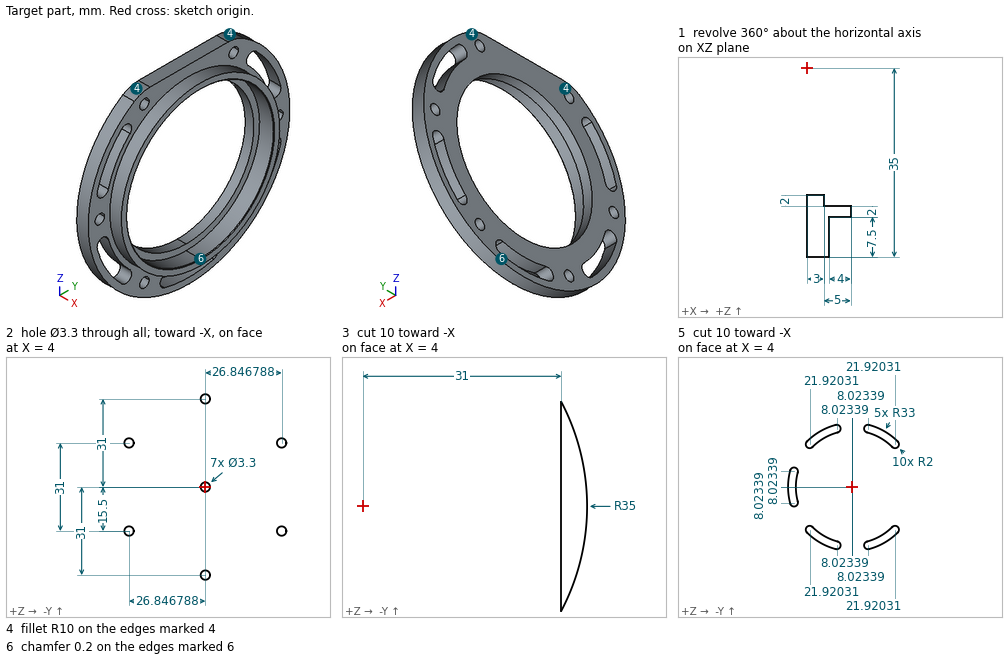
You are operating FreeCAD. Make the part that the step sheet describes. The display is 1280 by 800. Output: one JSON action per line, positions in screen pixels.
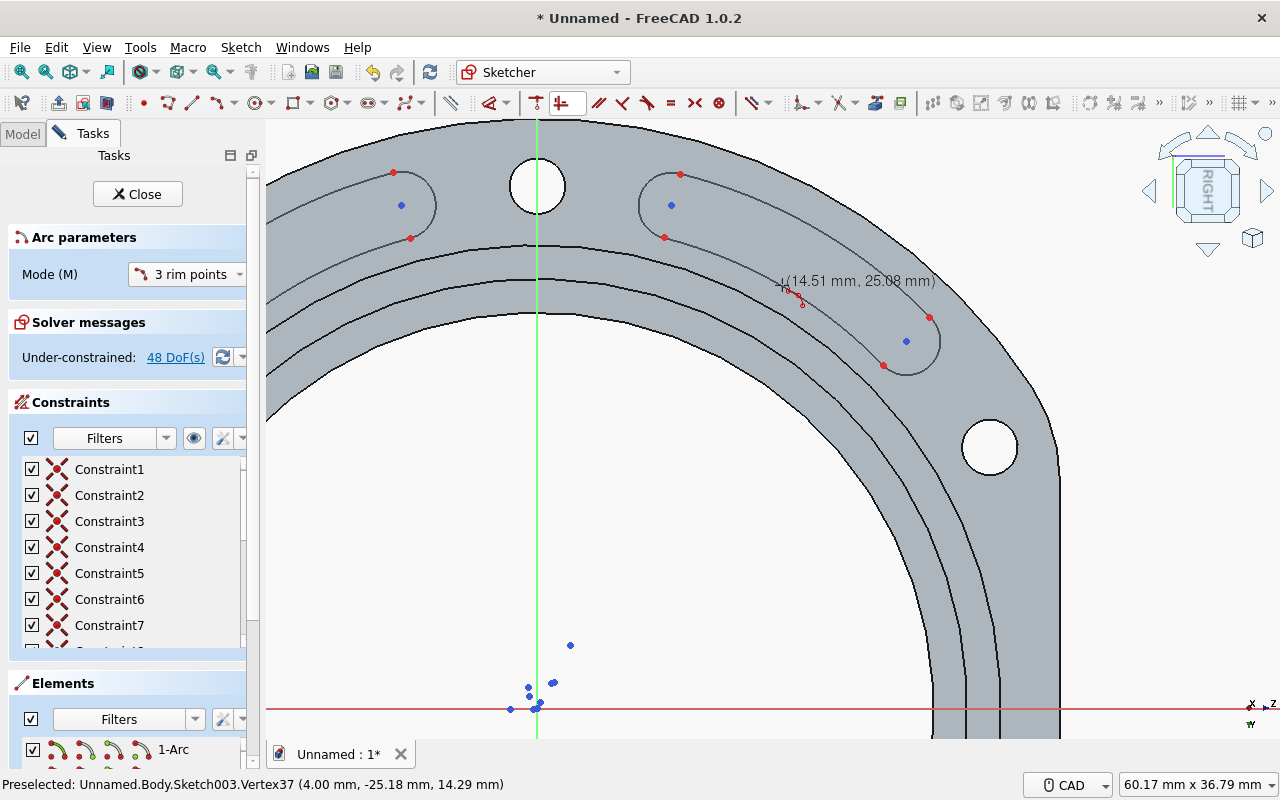
{"action": "scroll", "coordinate": [849, 266], "scroll_direction": "down", "scroll_amount": 5}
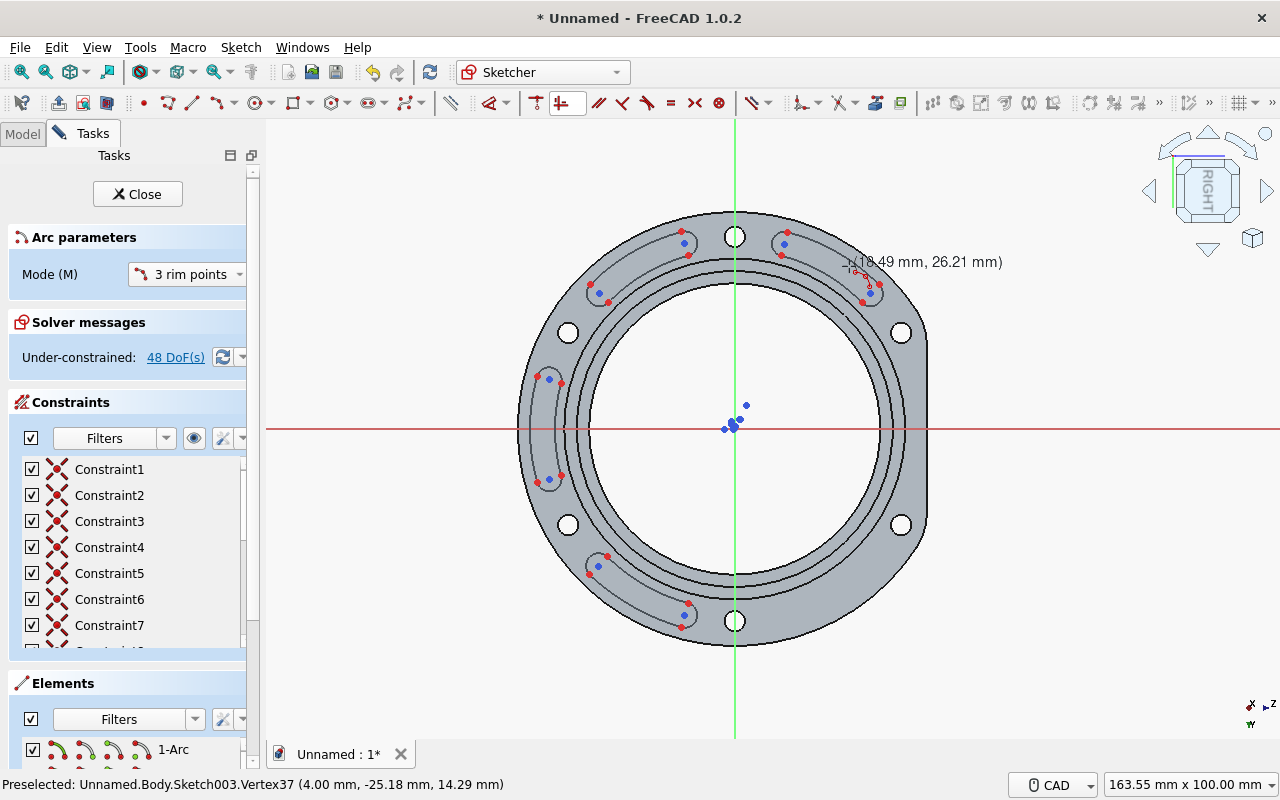
{"action": "left_click", "coordinate": [862, 556]}
{"action": "left_click", "coordinate": [781, 603]}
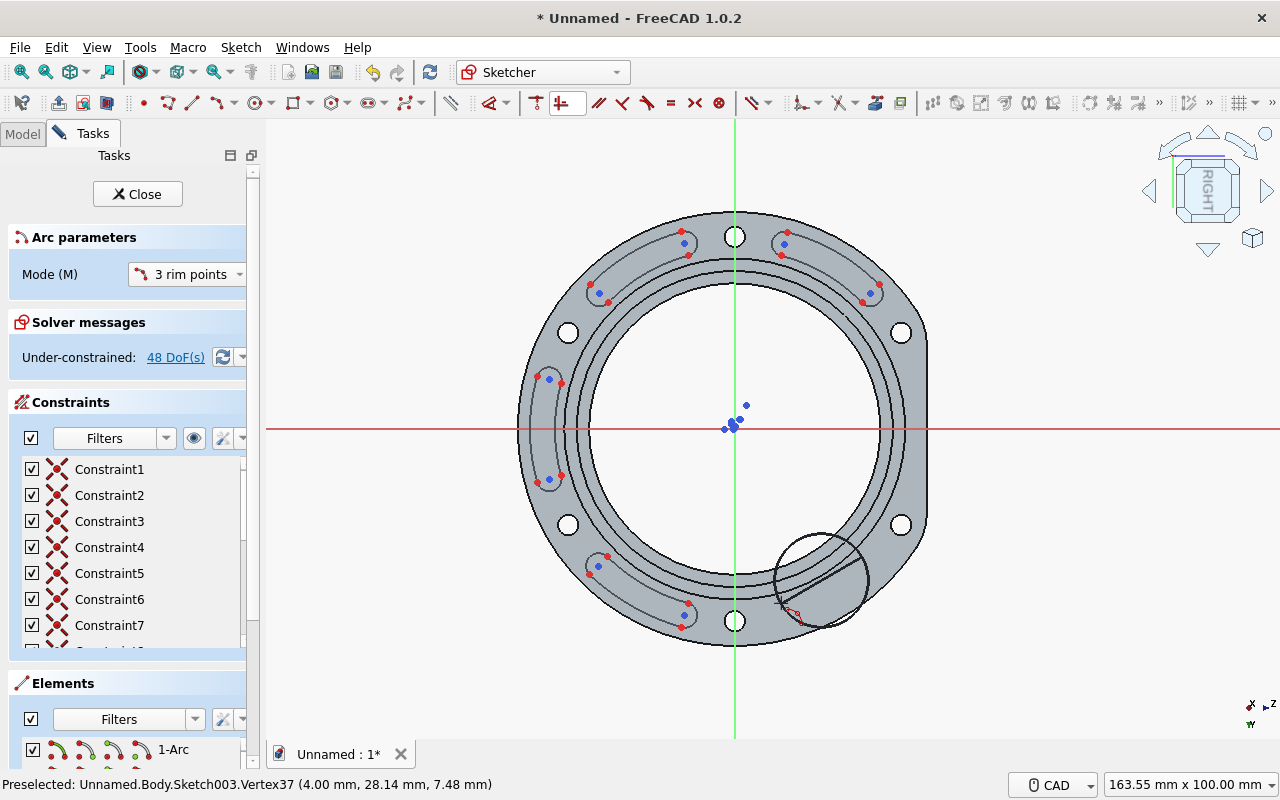
{"action": "scroll", "coordinate": [825, 585], "scroll_direction": "up", "scroll_amount": 5}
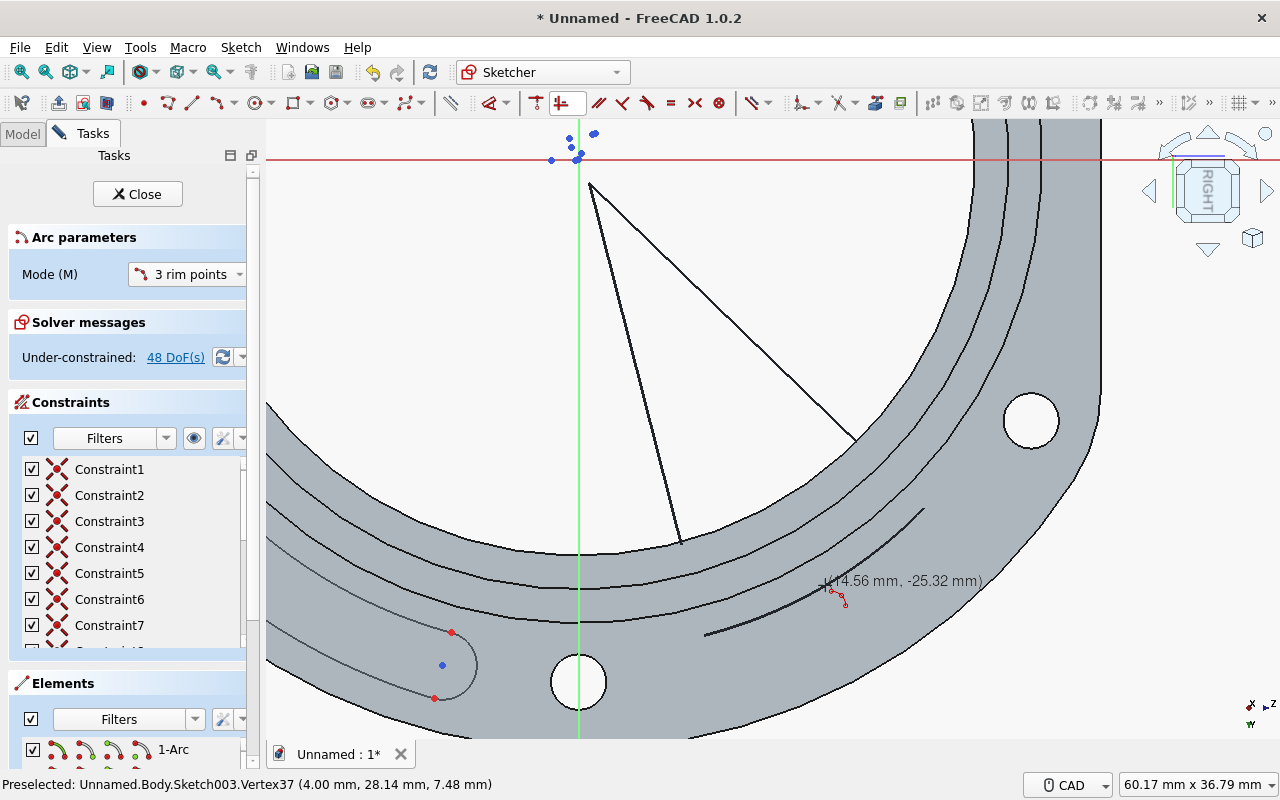
{"action": "left_click", "coordinate": [823, 583]}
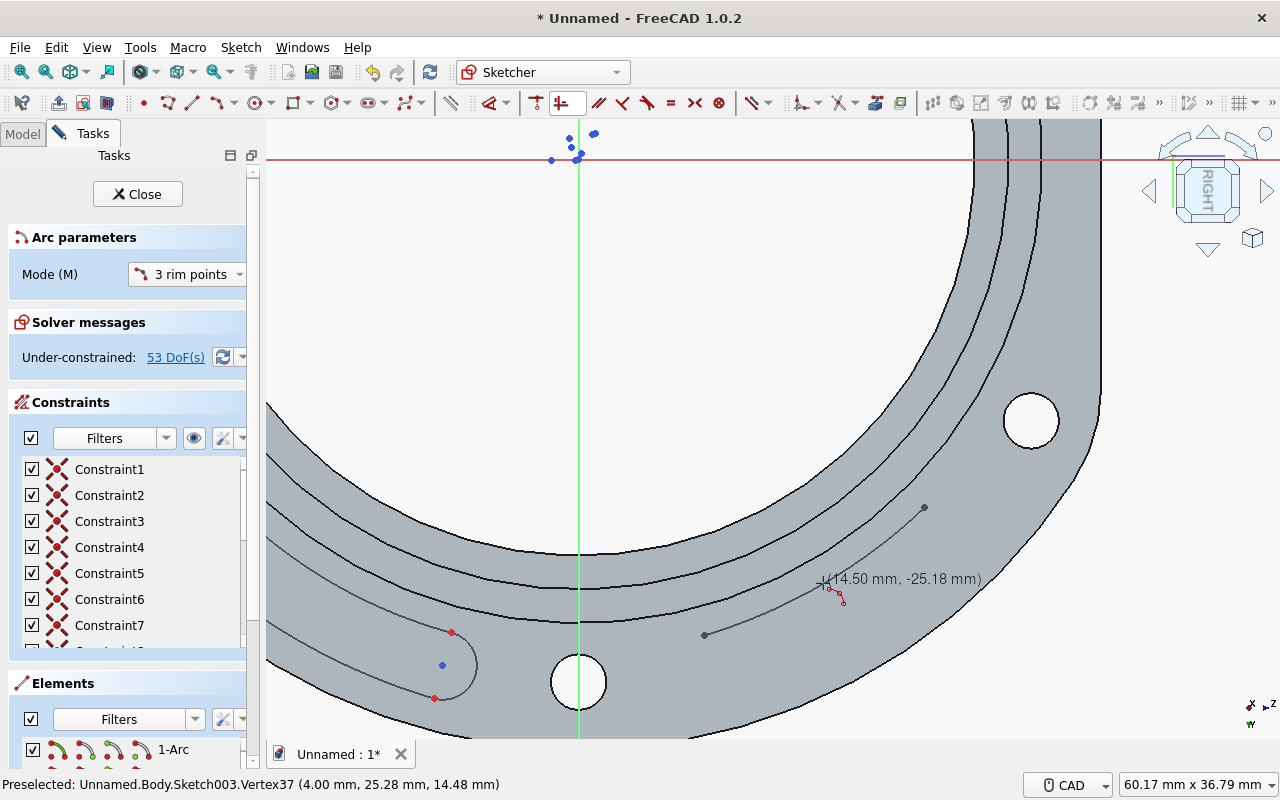
{"action": "left_click", "coordinate": [704, 635]}
{"action": "left_click", "coordinate": [723, 697]}
{"action": "left_click", "coordinate": [681, 673]}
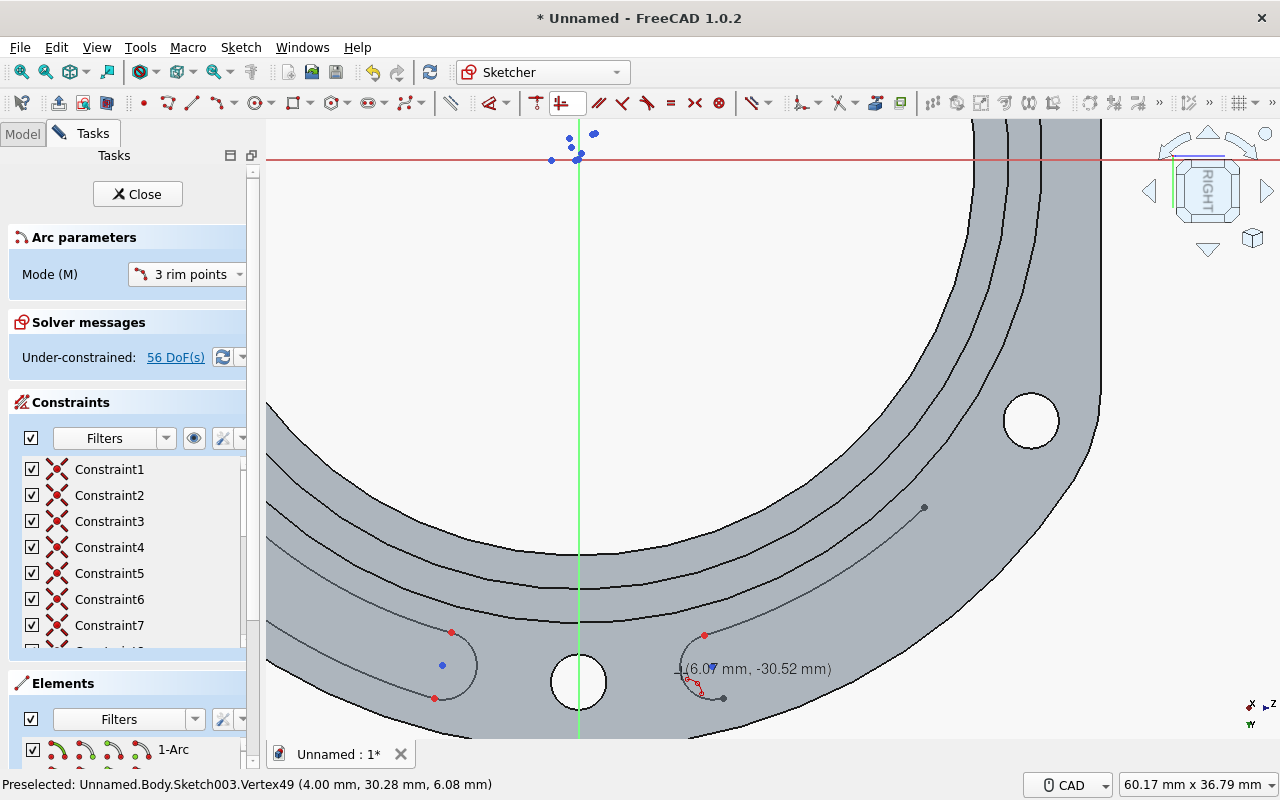
{"action": "left_click", "coordinate": [723, 698]}
{"action": "left_click", "coordinate": [972, 553]}
{"action": "left_click", "coordinate": [857, 641]}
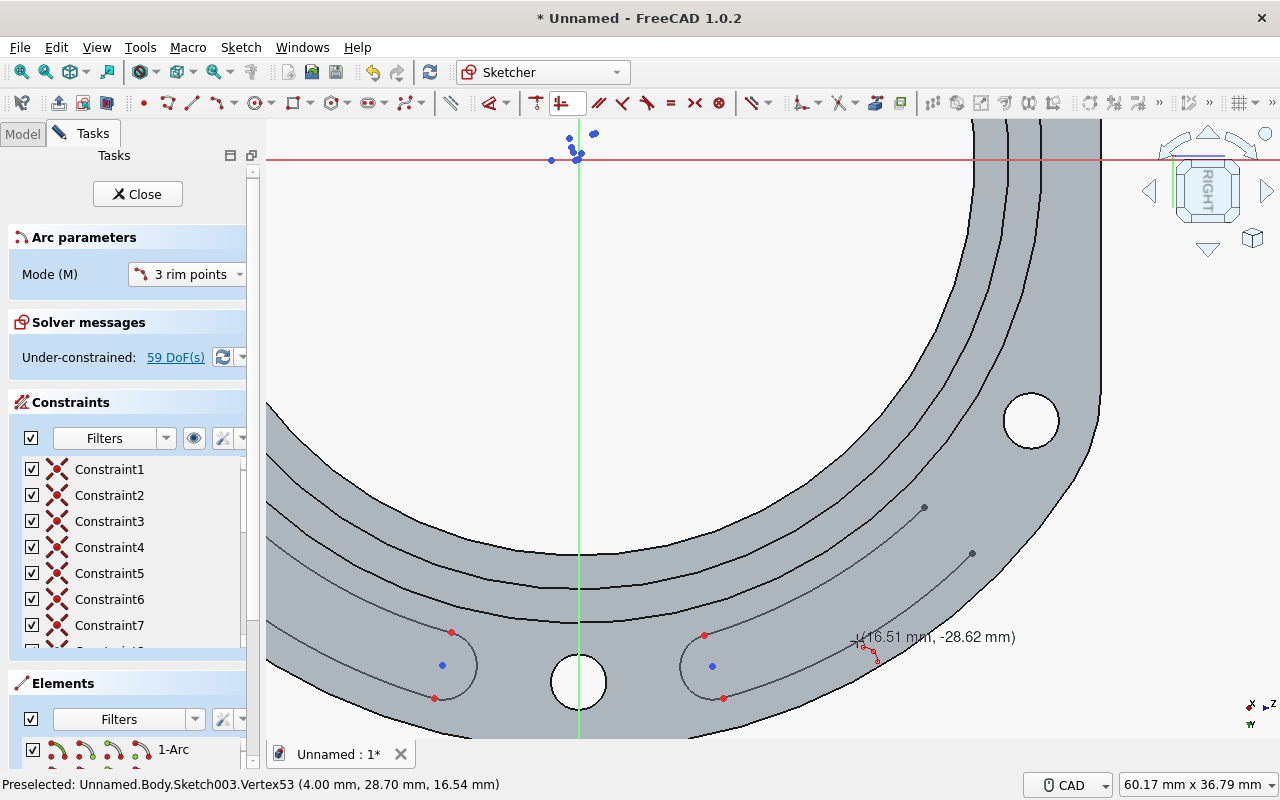
{"action": "left_click", "coordinate": [972, 554]}
{"action": "left_click", "coordinate": [925, 508]}
{"action": "left_click", "coordinate": [972, 505]}
{"action": "key", "text": "Escape"}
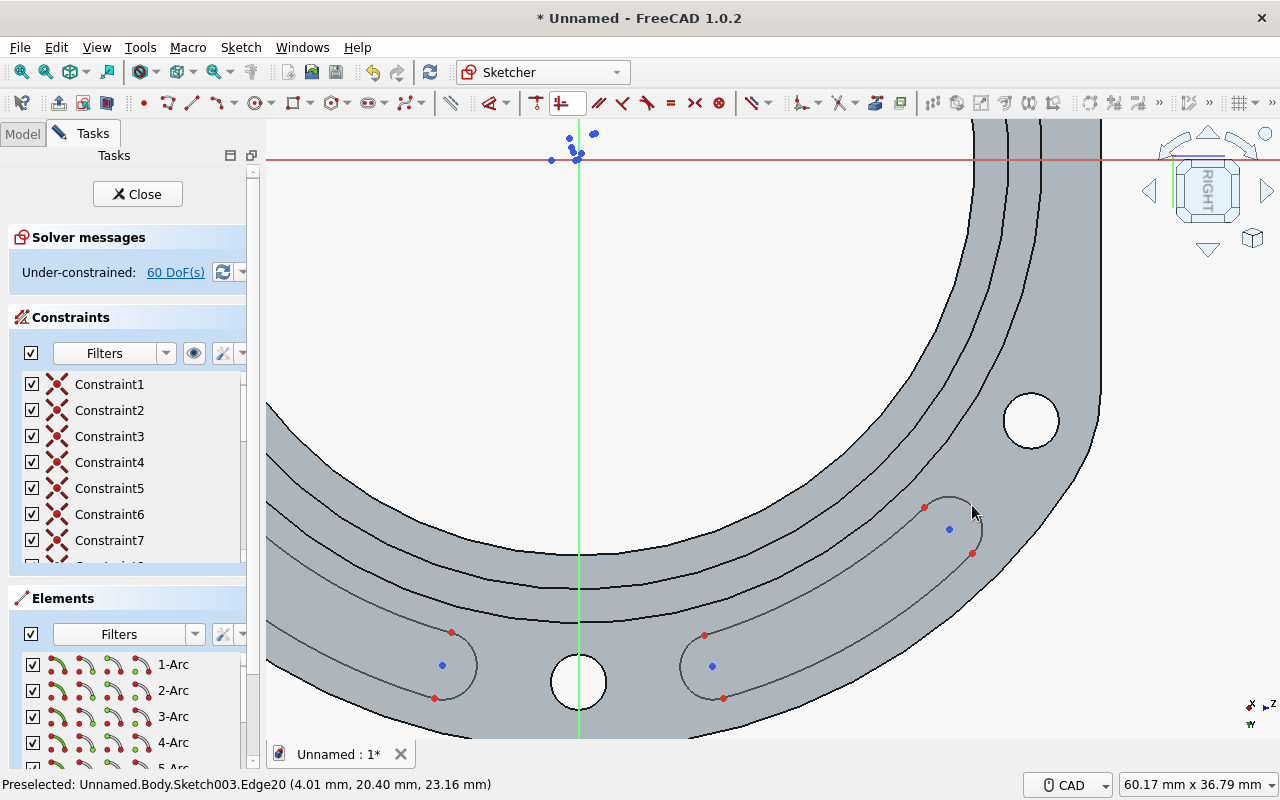
{"action": "scroll", "coordinate": [825, 586], "scroll_direction": "down", "scroll_amount": 5}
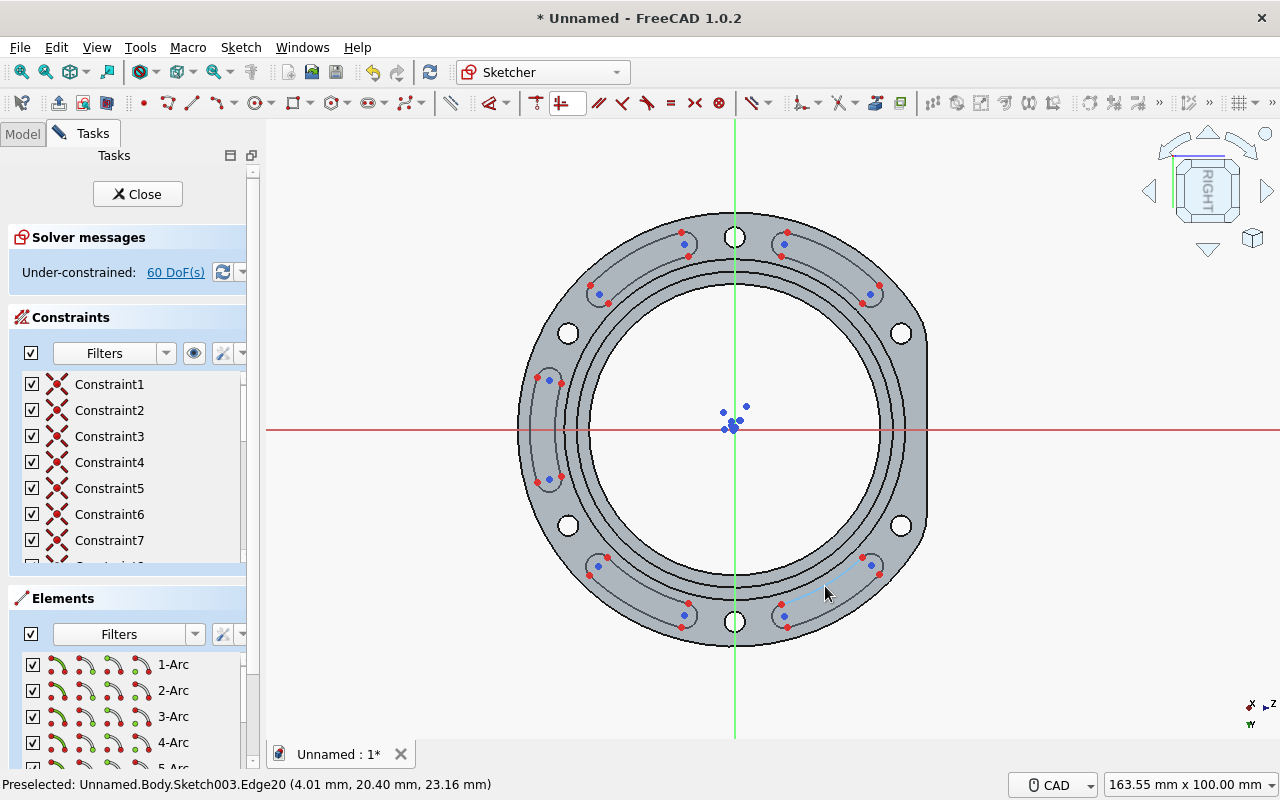
{"action": "left_click", "coordinate": [597, 554]}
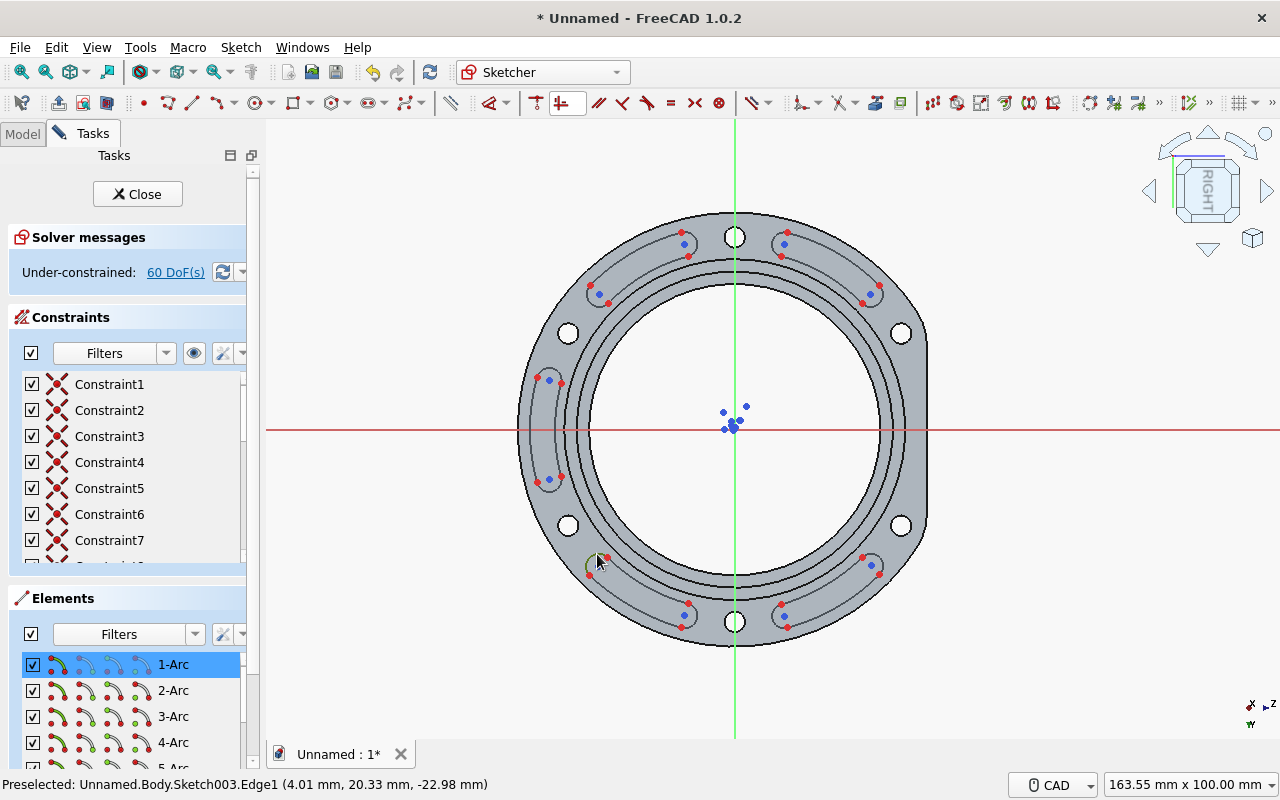
{"action": "left_click", "coordinate": [615, 596]}